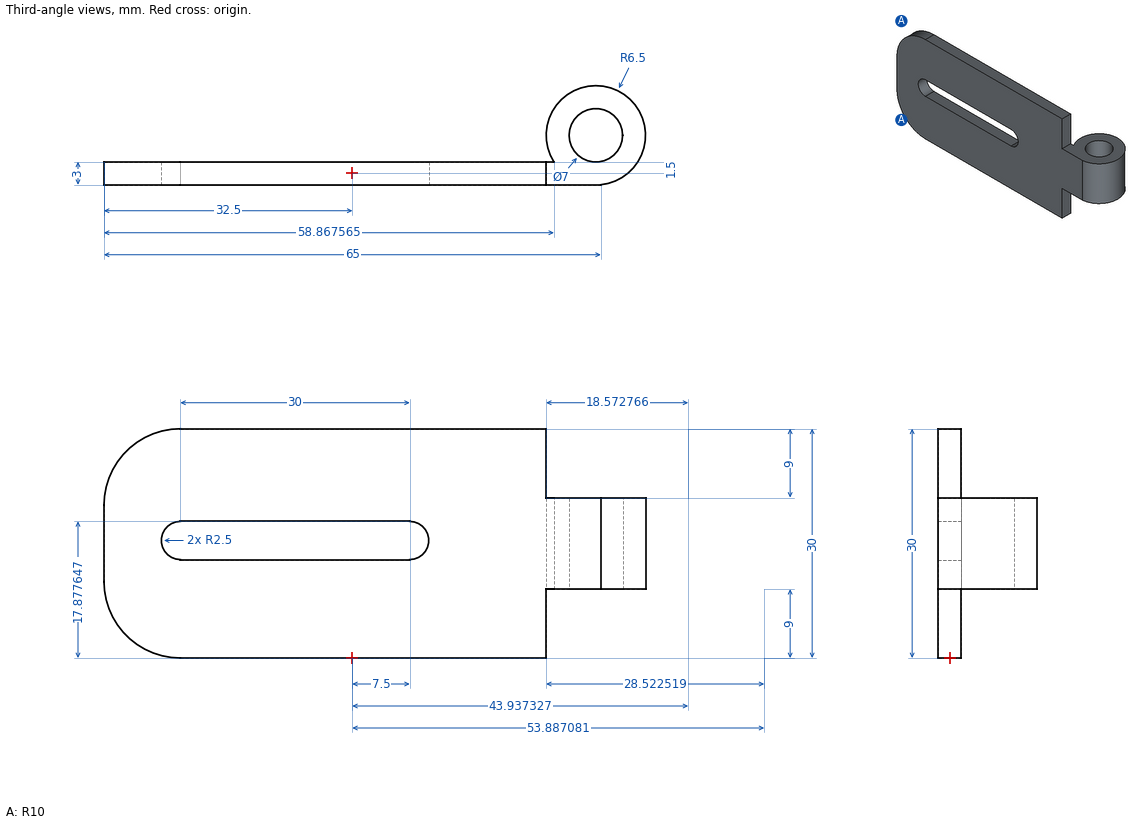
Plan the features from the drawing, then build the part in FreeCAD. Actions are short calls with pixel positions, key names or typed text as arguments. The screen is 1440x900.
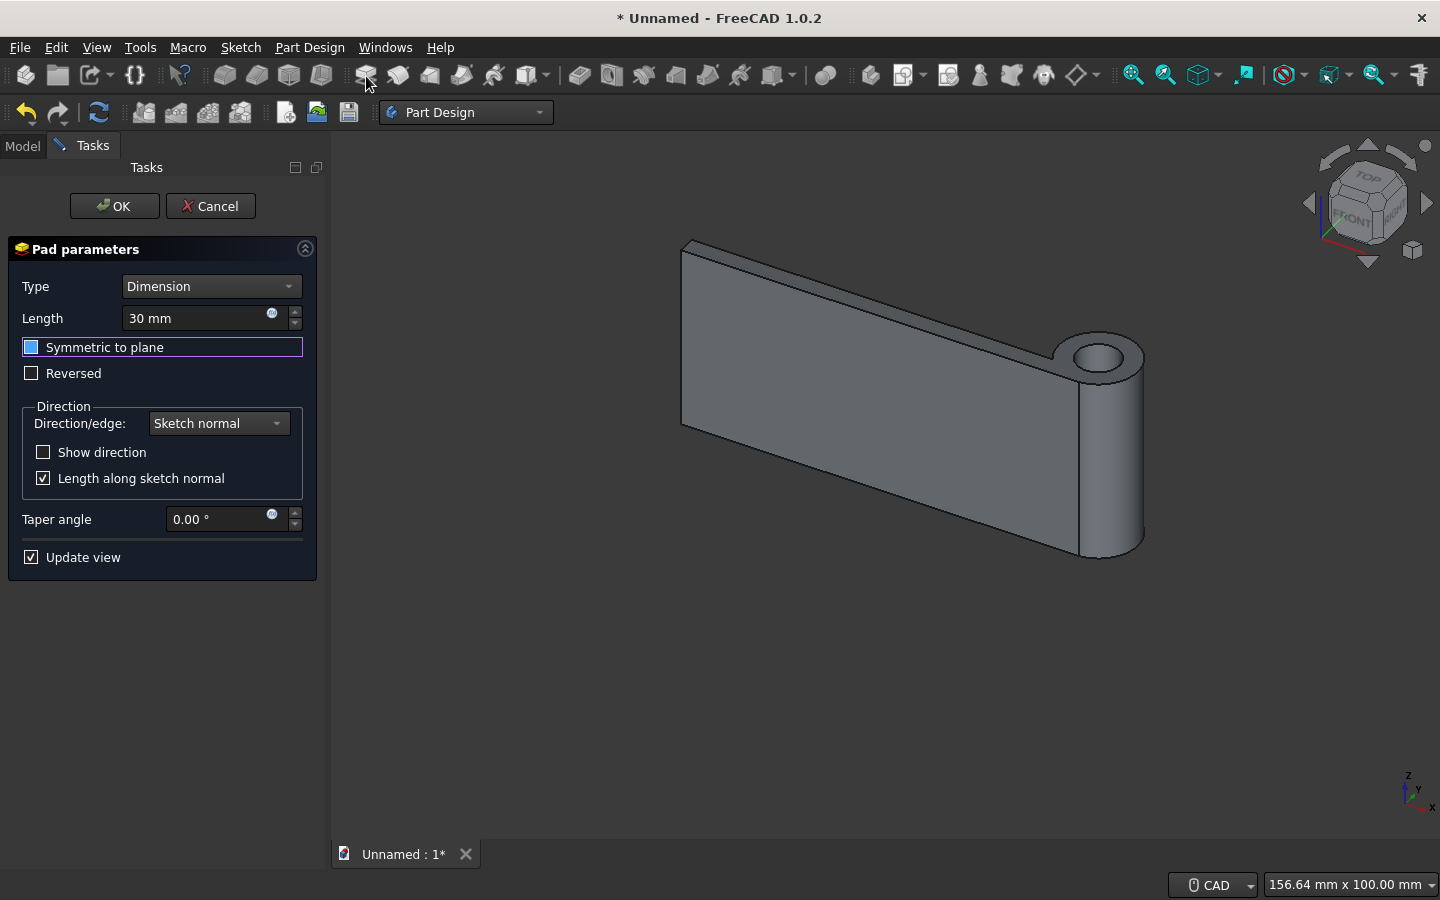
click(115, 206)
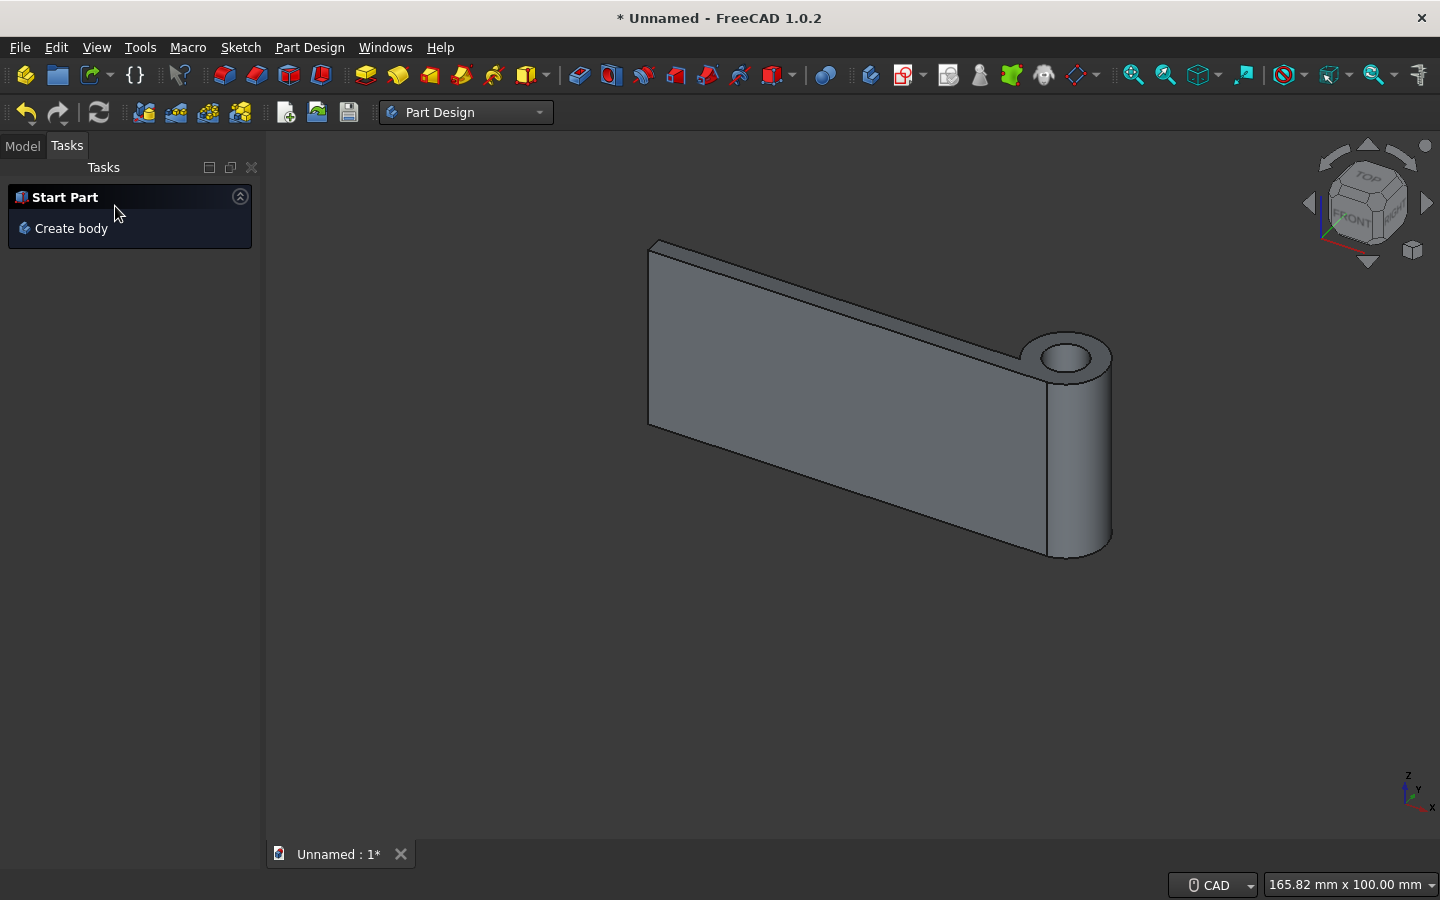
scroll(654, 244, up, 4)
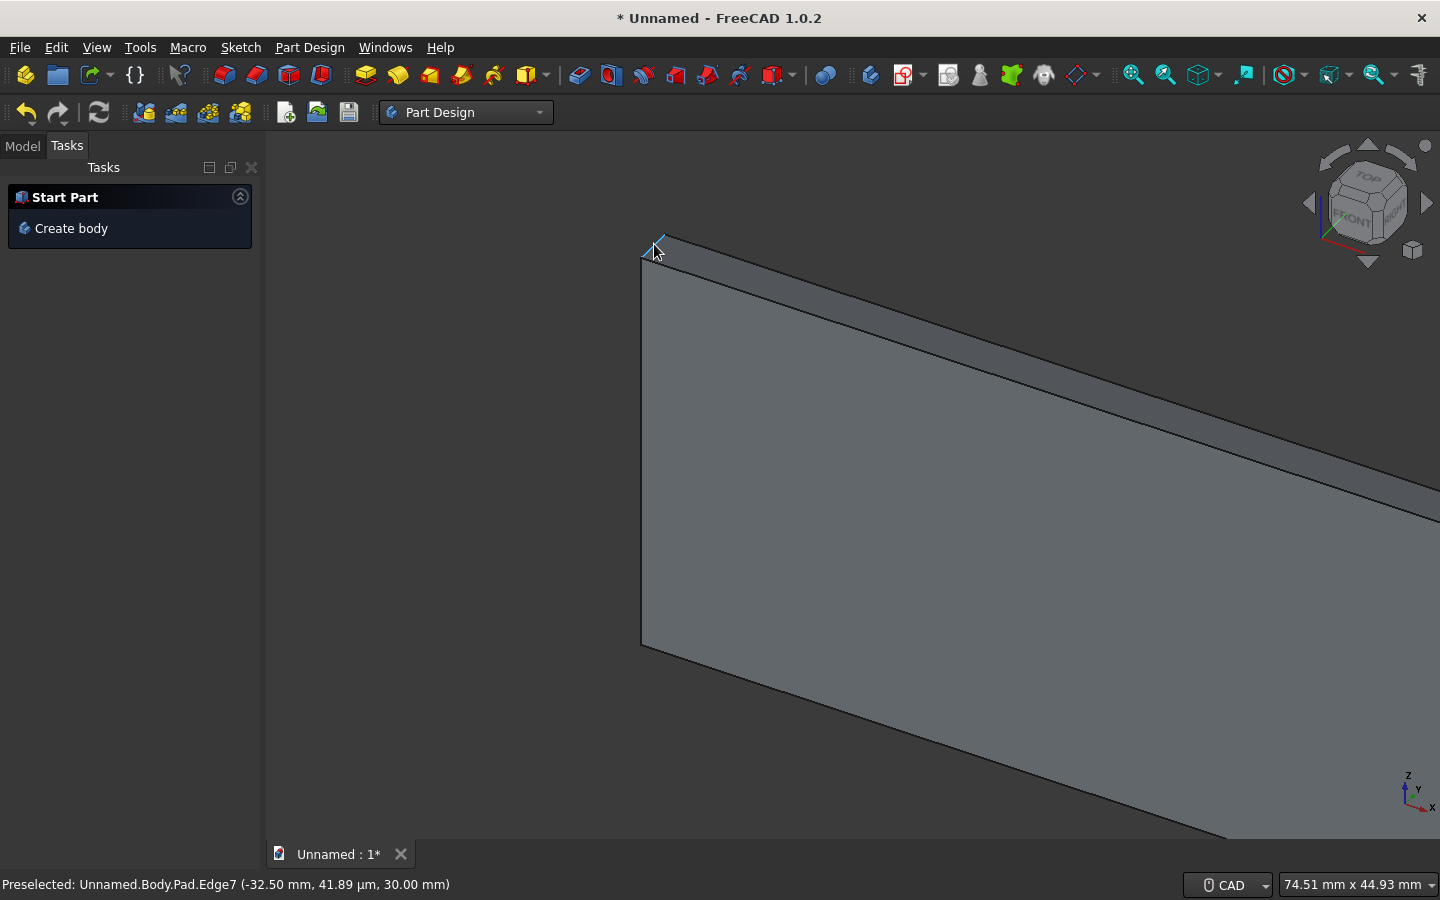
click(1134, 76)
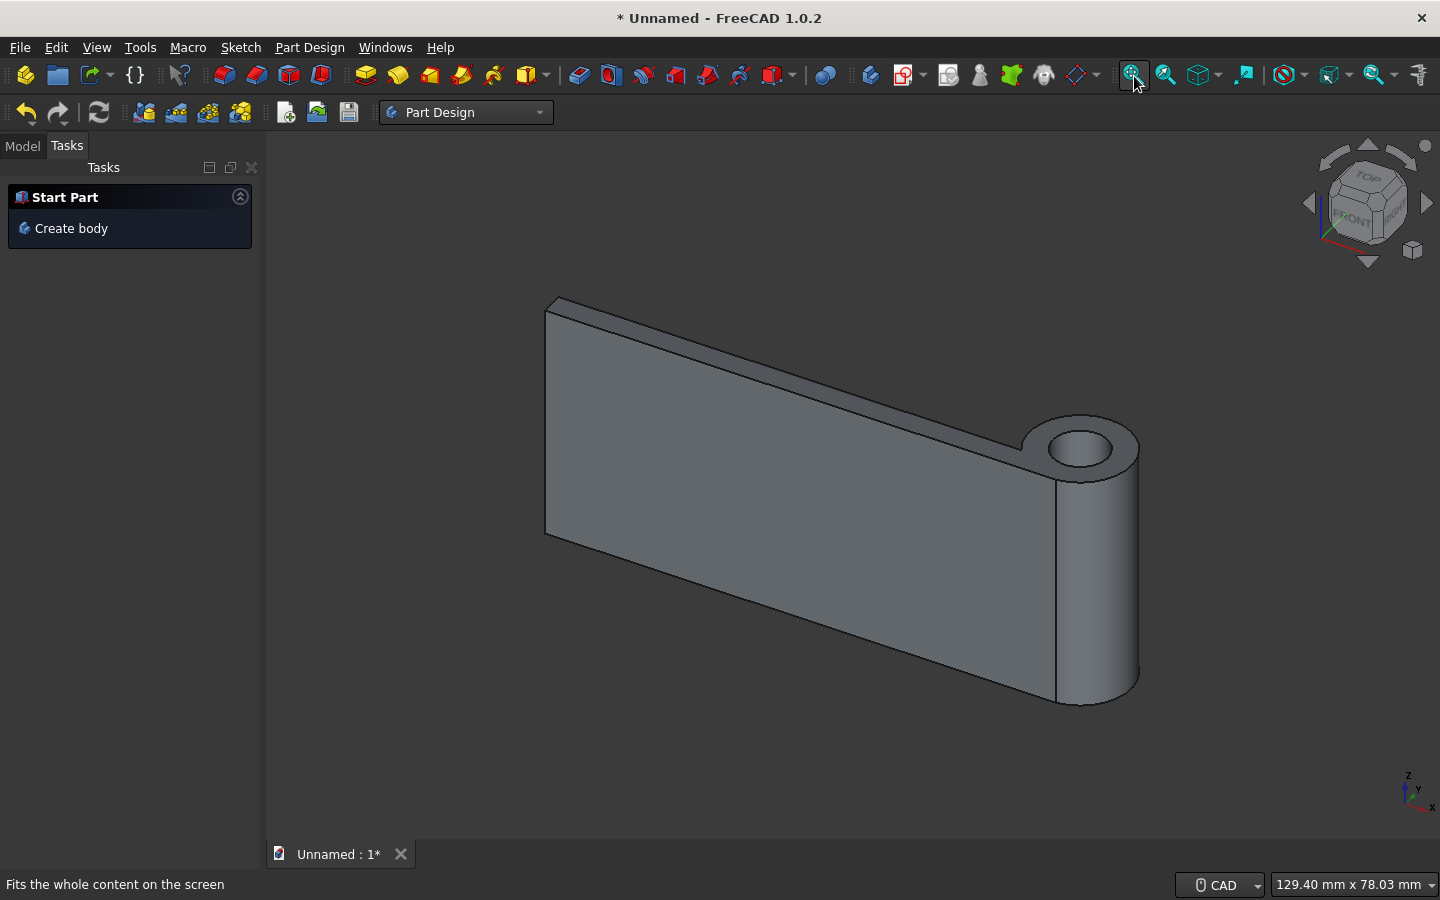
key(0)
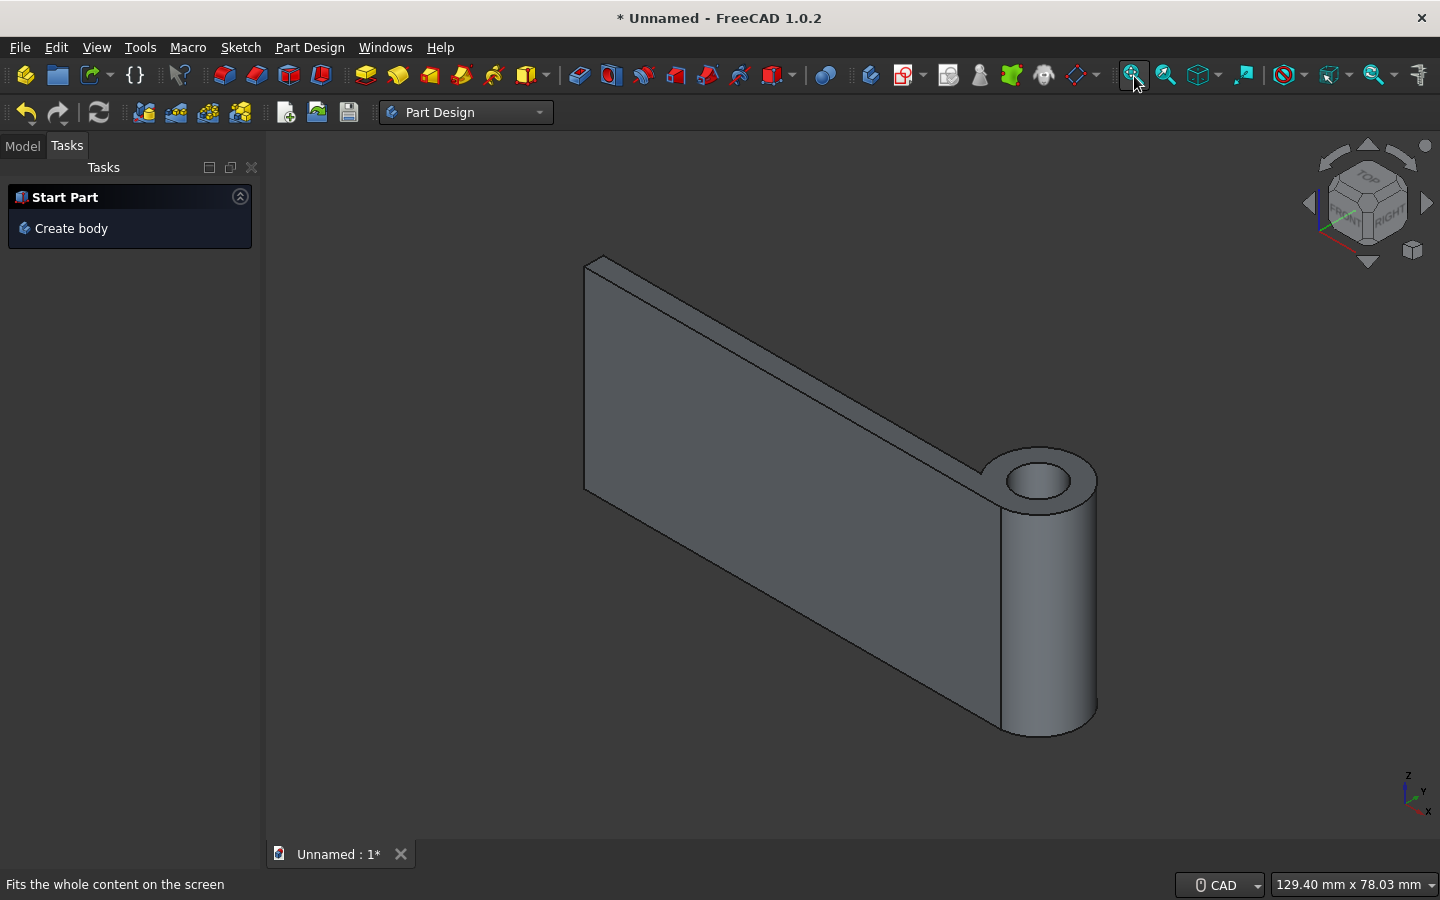
key(2)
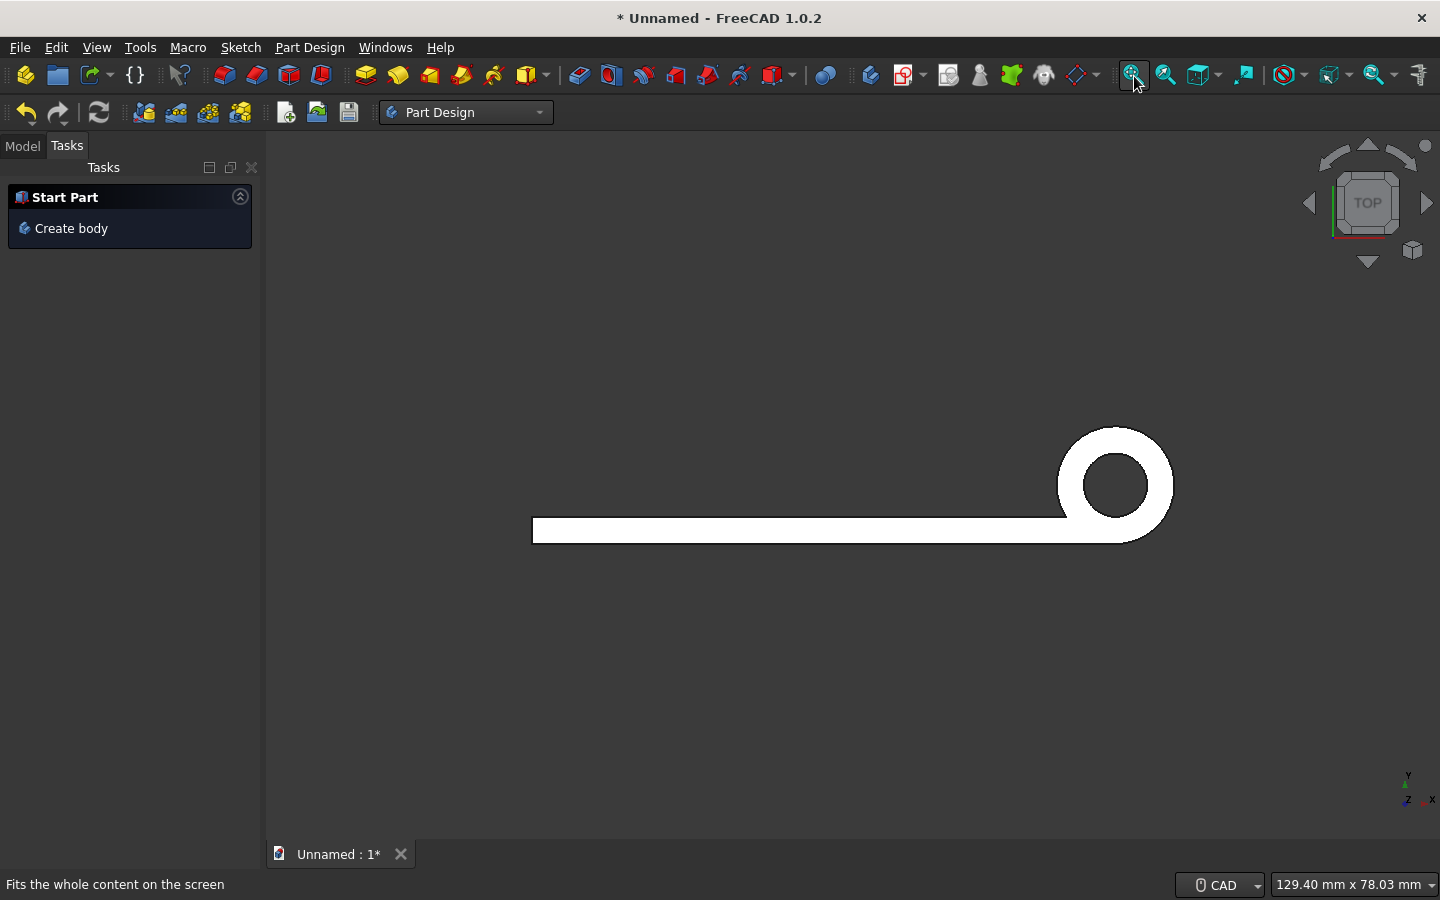
click(532, 529)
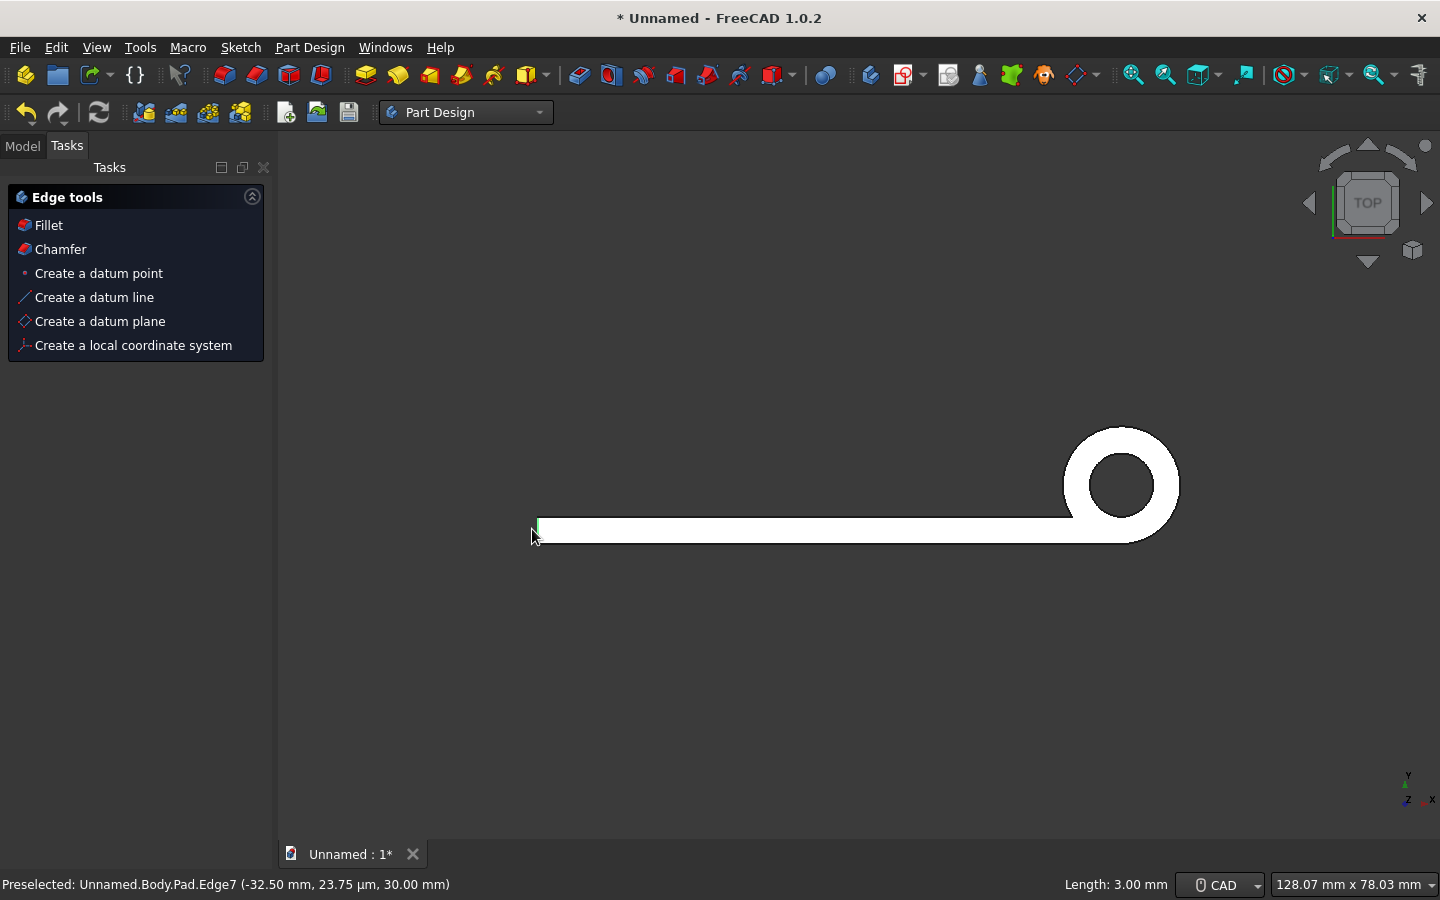
key(1)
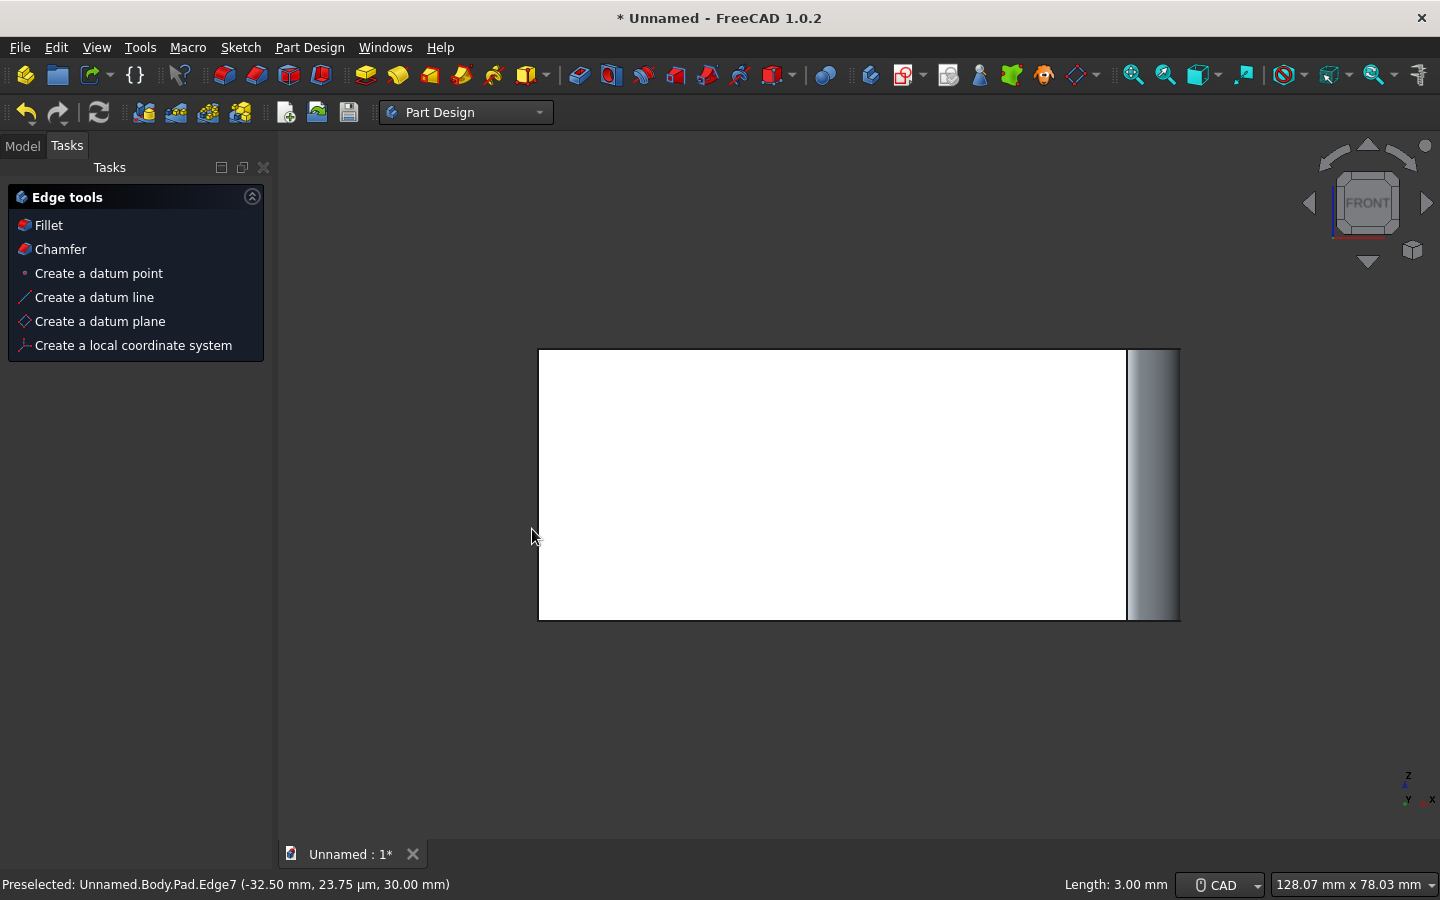
key(3)